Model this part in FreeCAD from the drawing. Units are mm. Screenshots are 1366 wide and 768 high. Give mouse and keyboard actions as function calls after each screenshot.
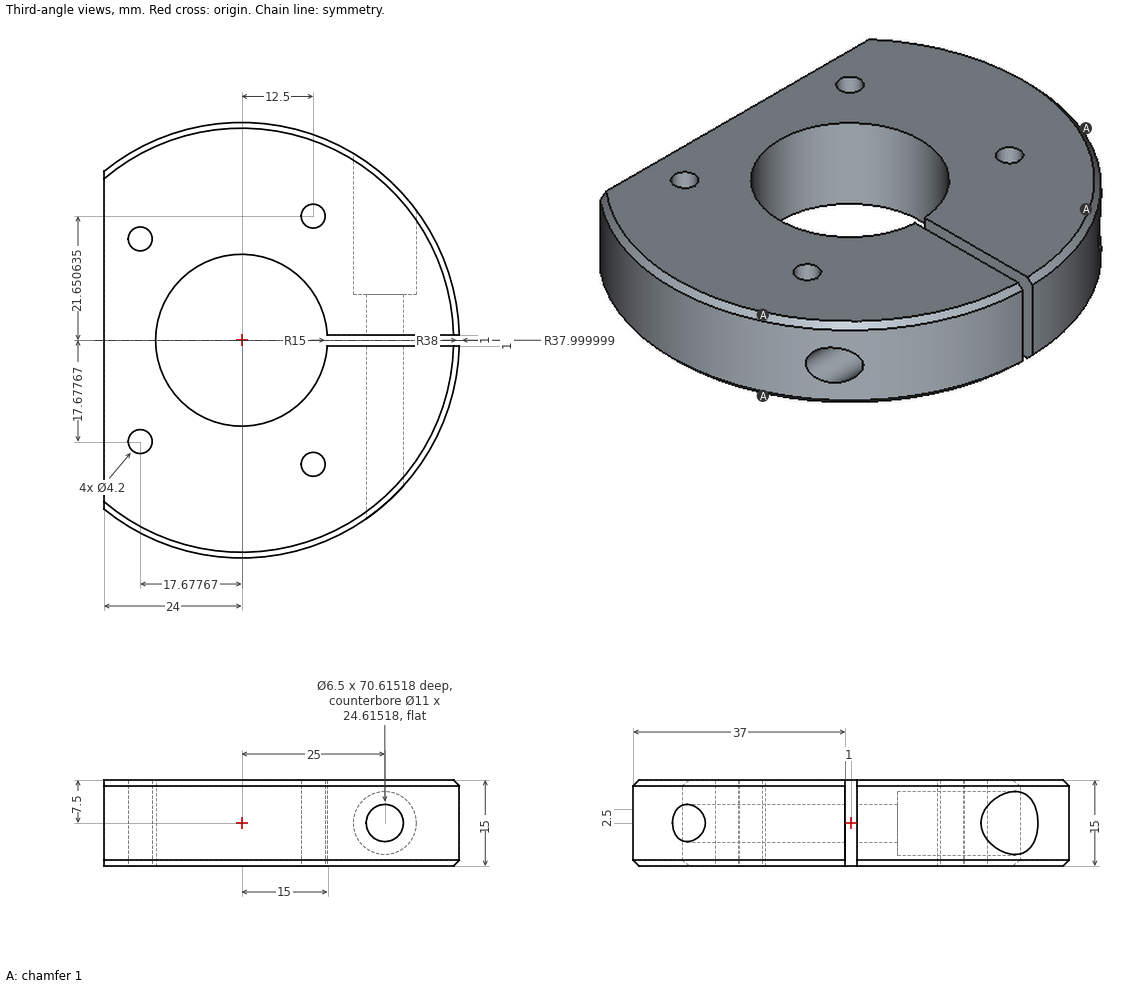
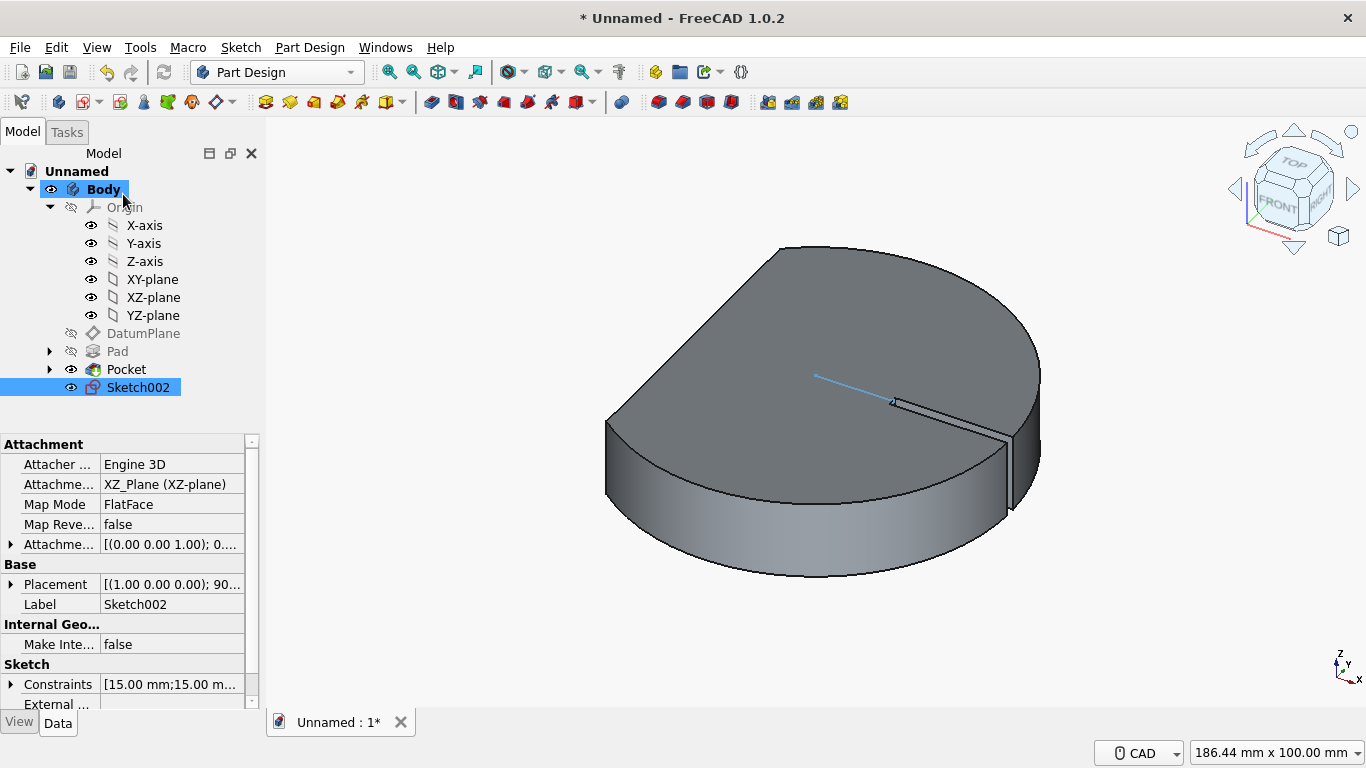
click(480, 102)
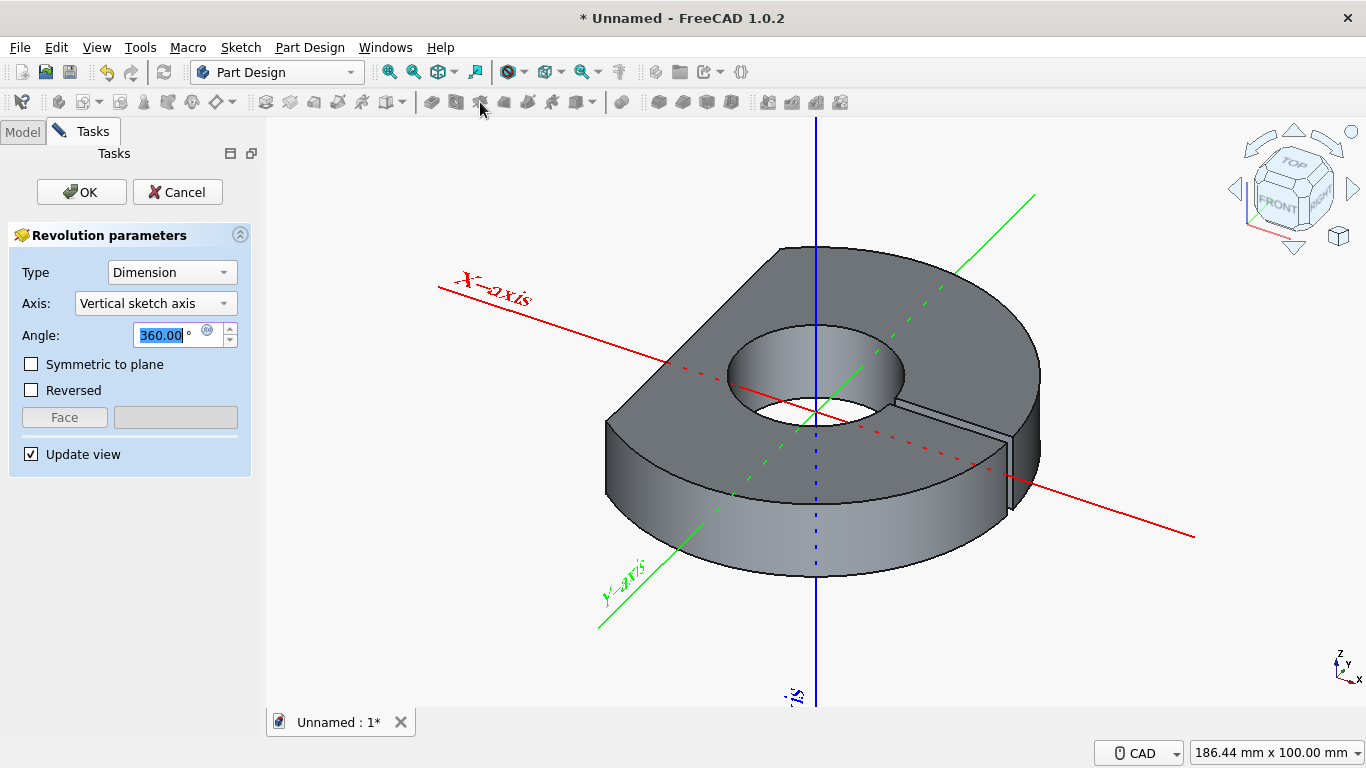
click(82, 192)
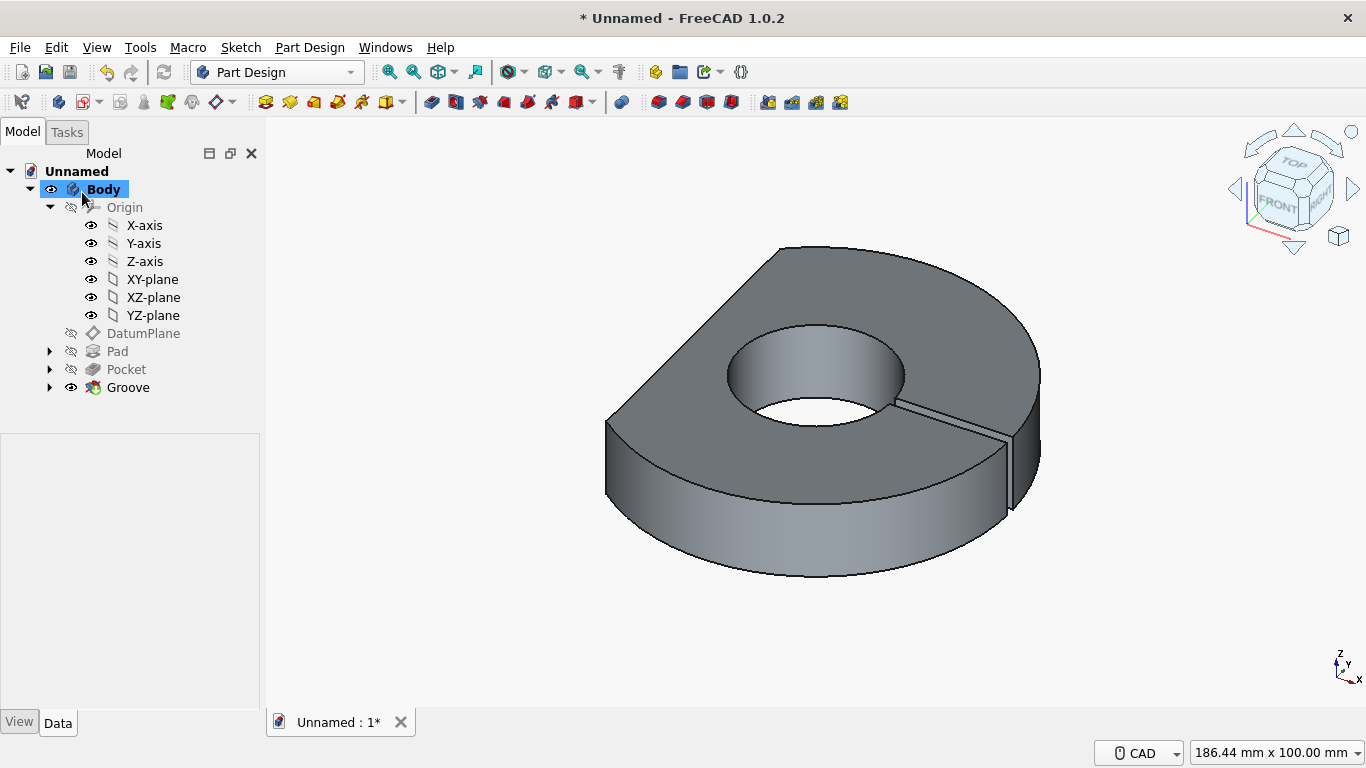
click(961, 338)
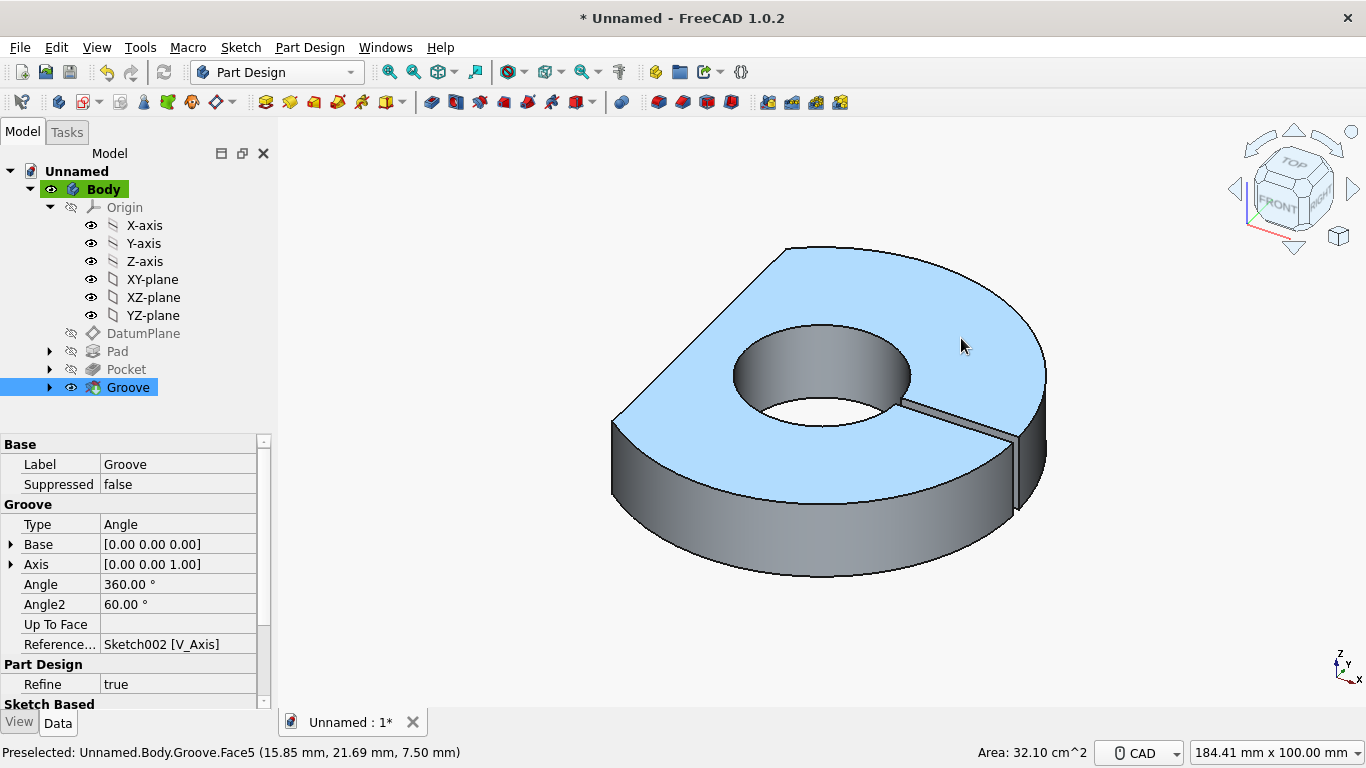
click(84, 102)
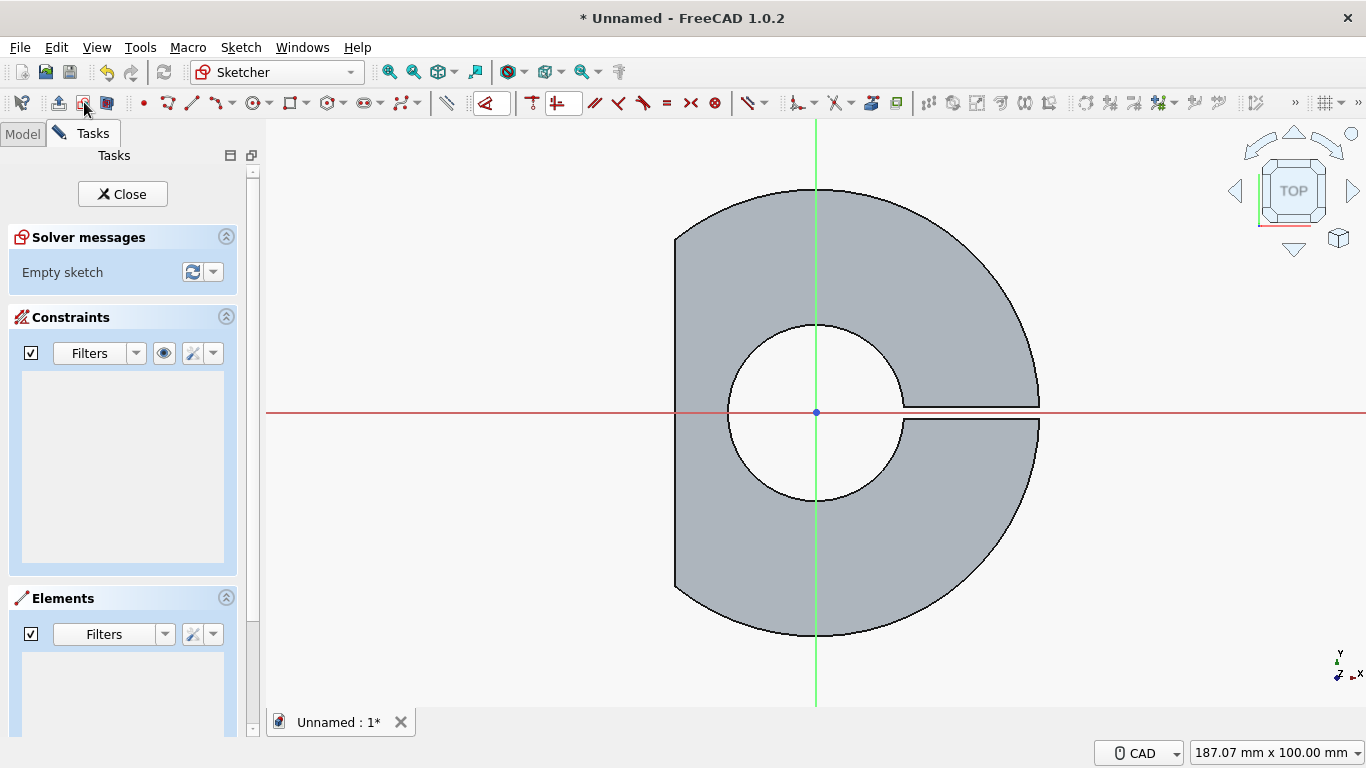
click(254, 104)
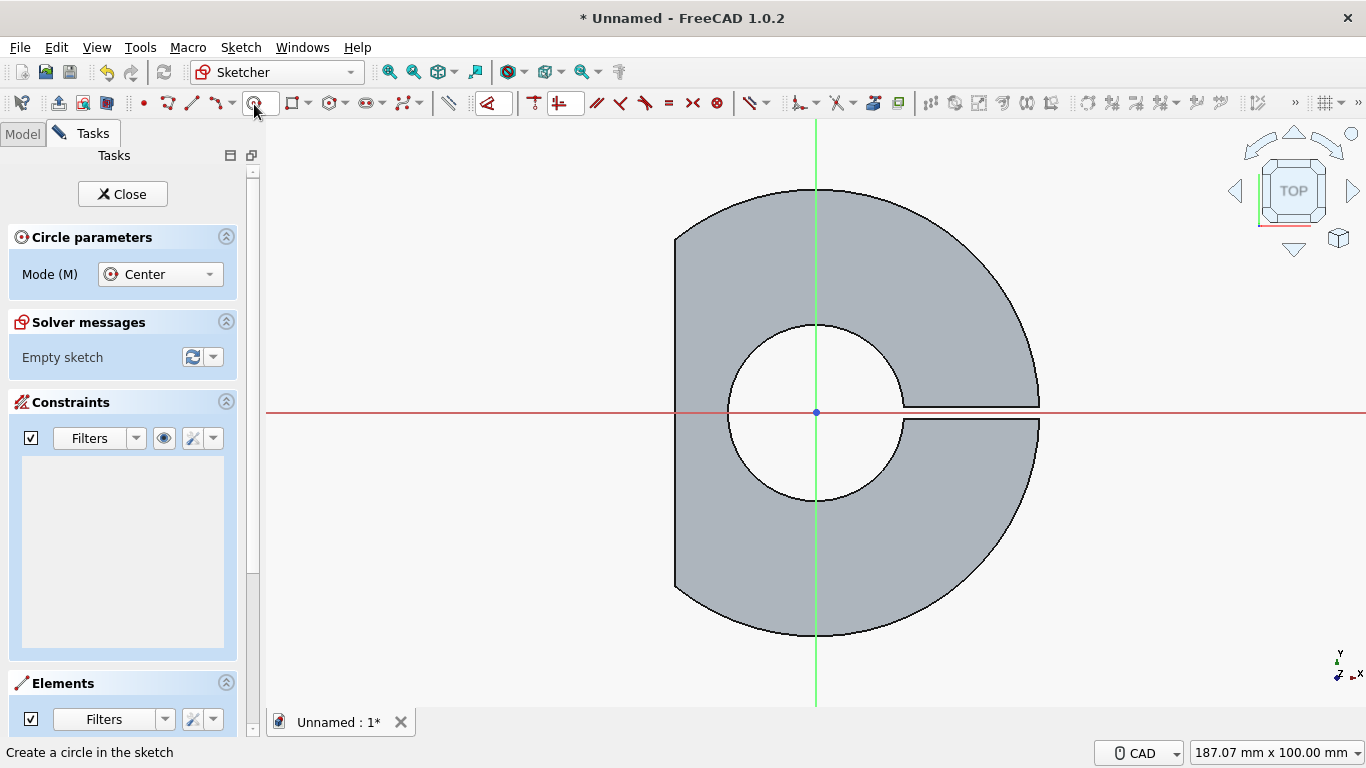
scroll(712, 517, up, 4)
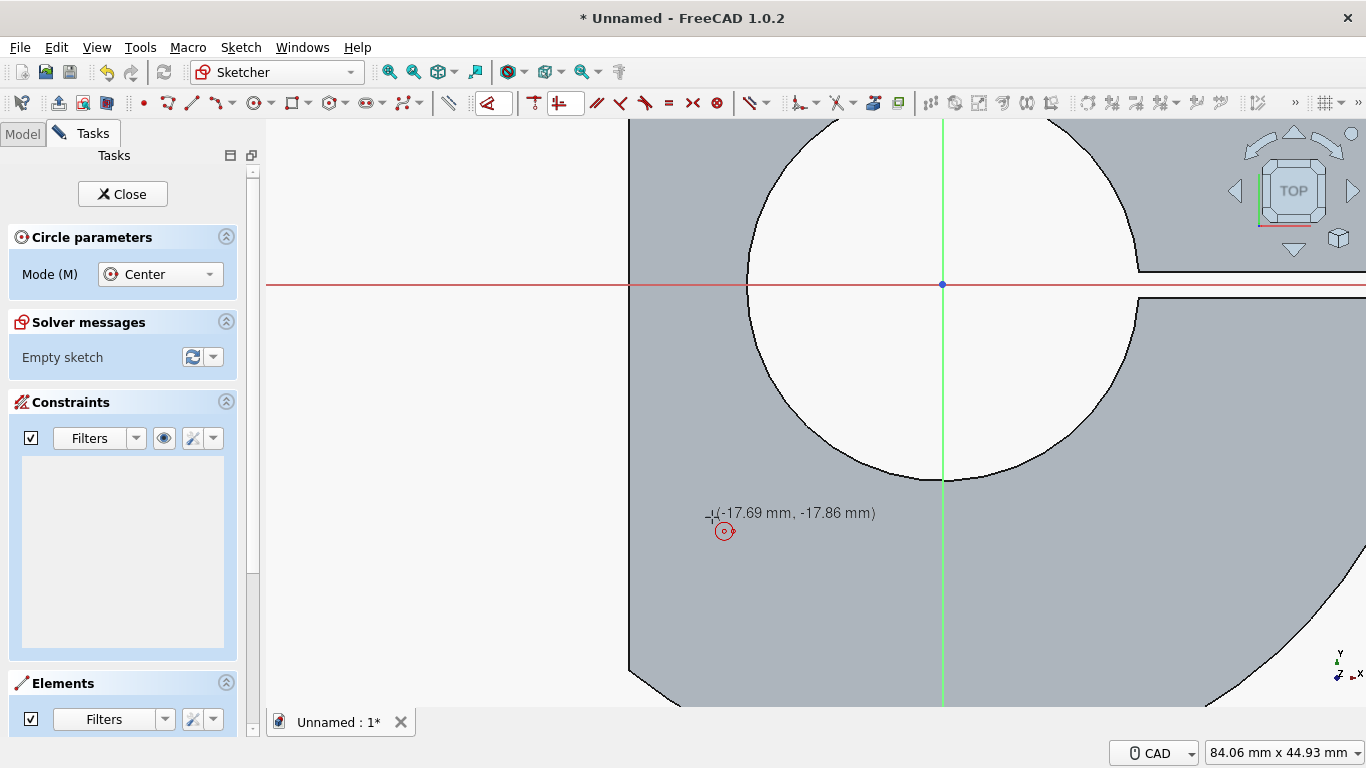
click(712, 516)
move(731, 497)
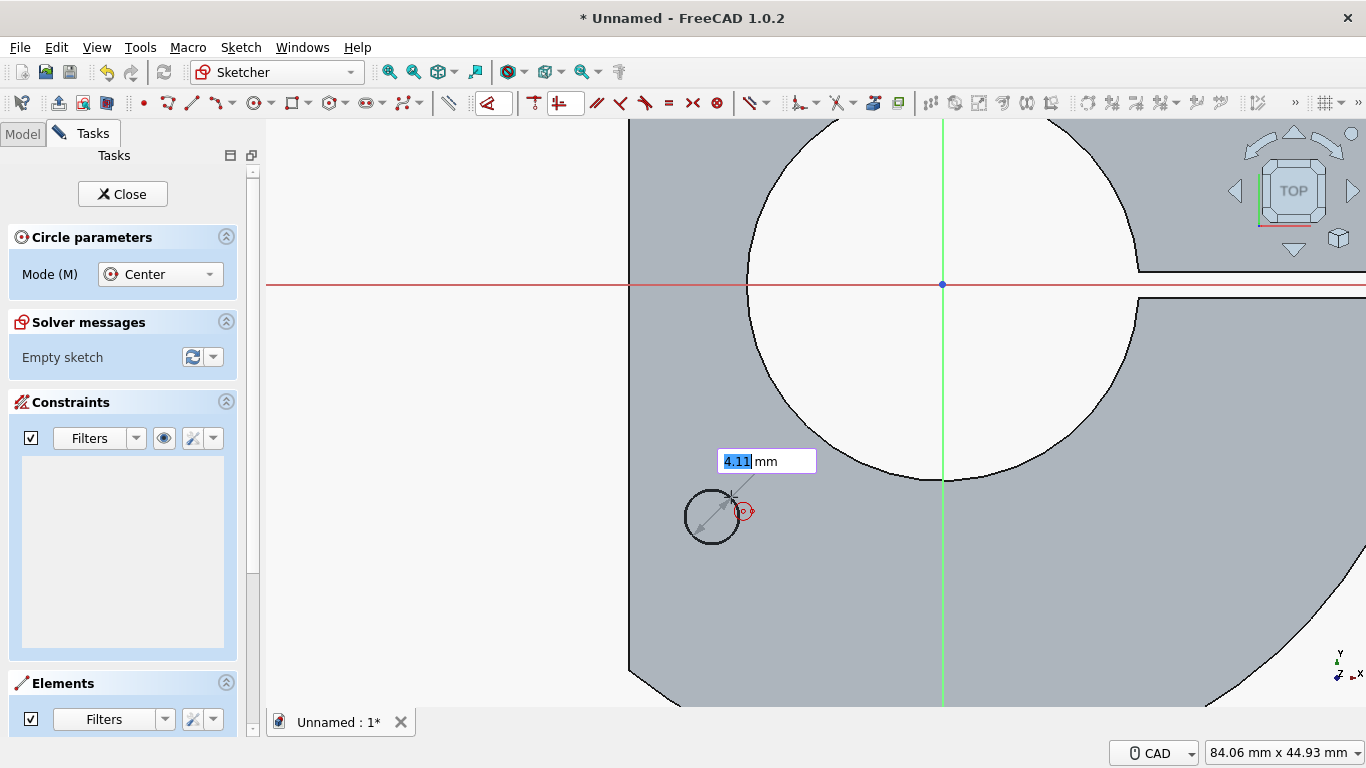
text(4.2)
key(Return)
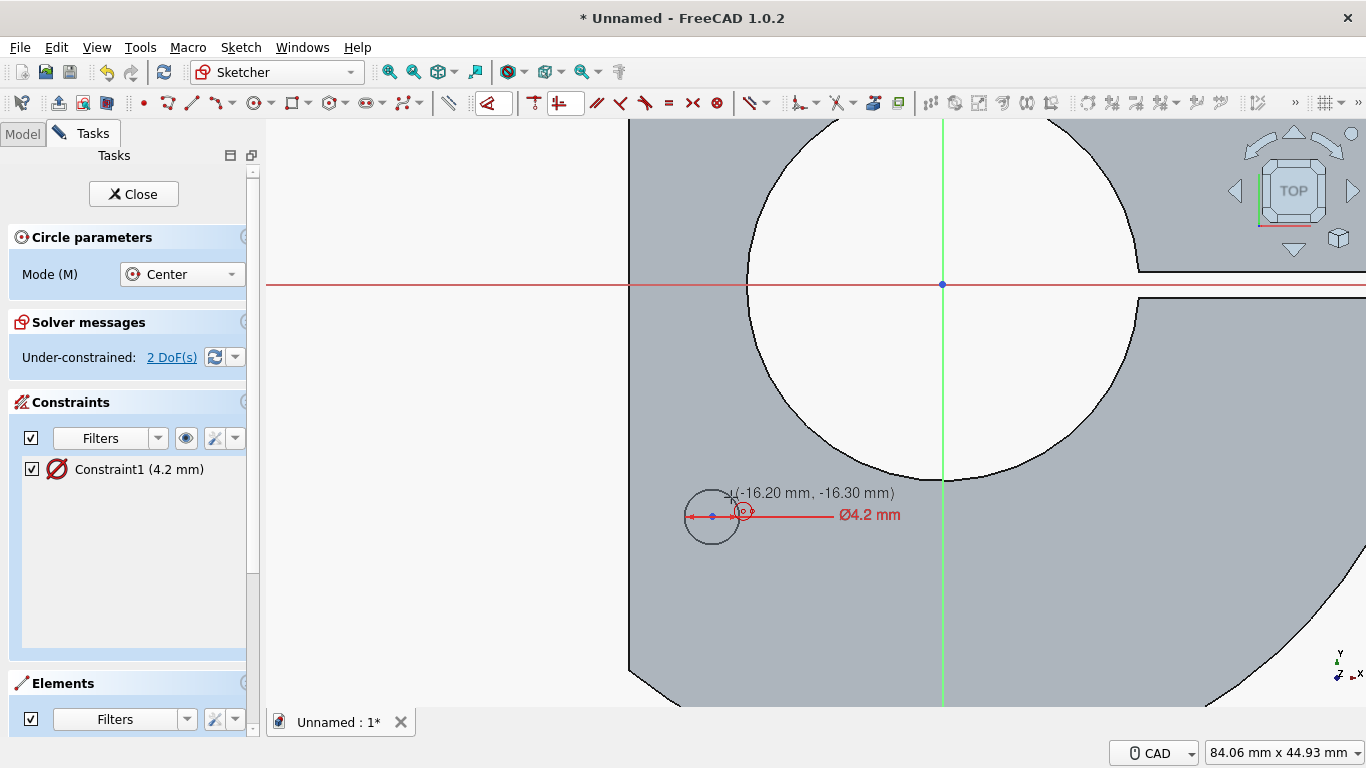
scroll(551, 569, down, 3)